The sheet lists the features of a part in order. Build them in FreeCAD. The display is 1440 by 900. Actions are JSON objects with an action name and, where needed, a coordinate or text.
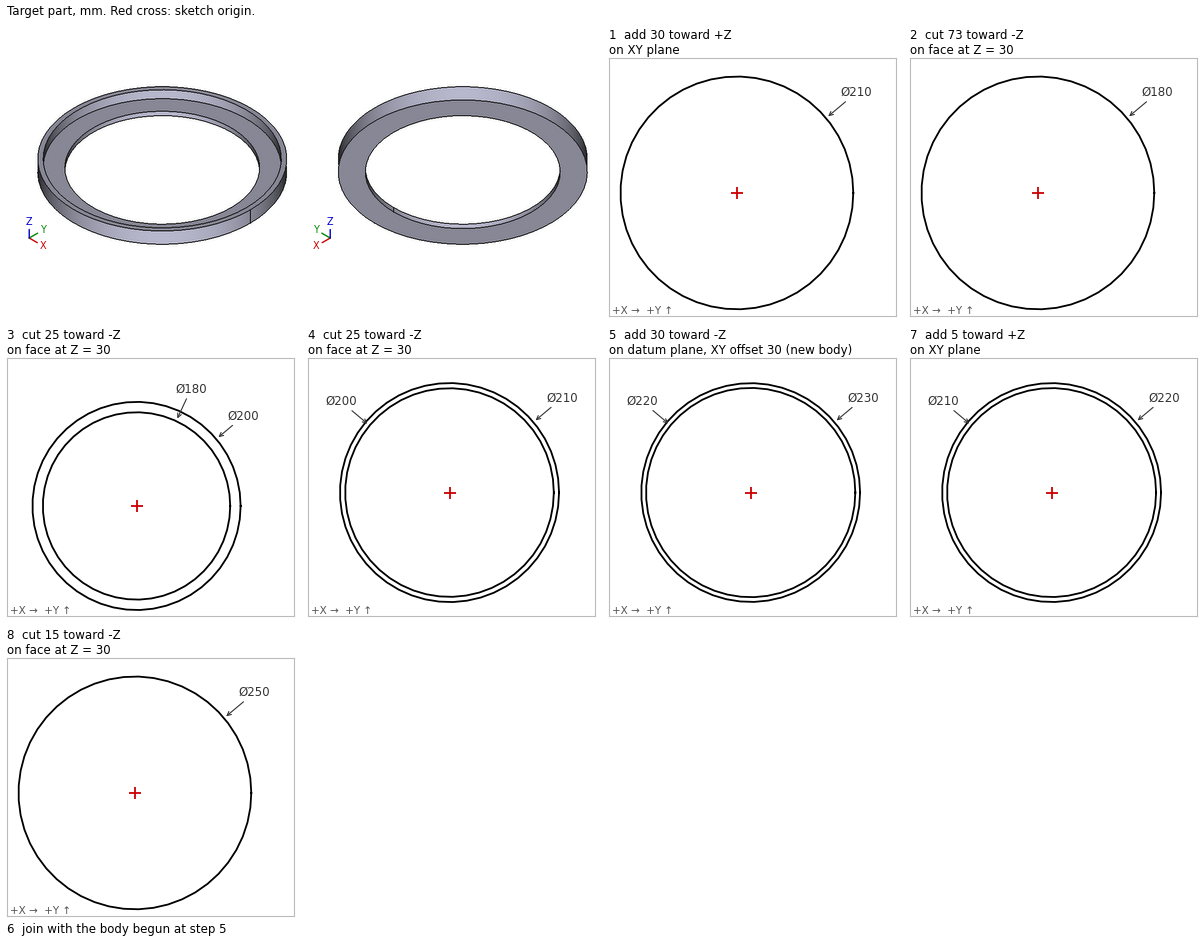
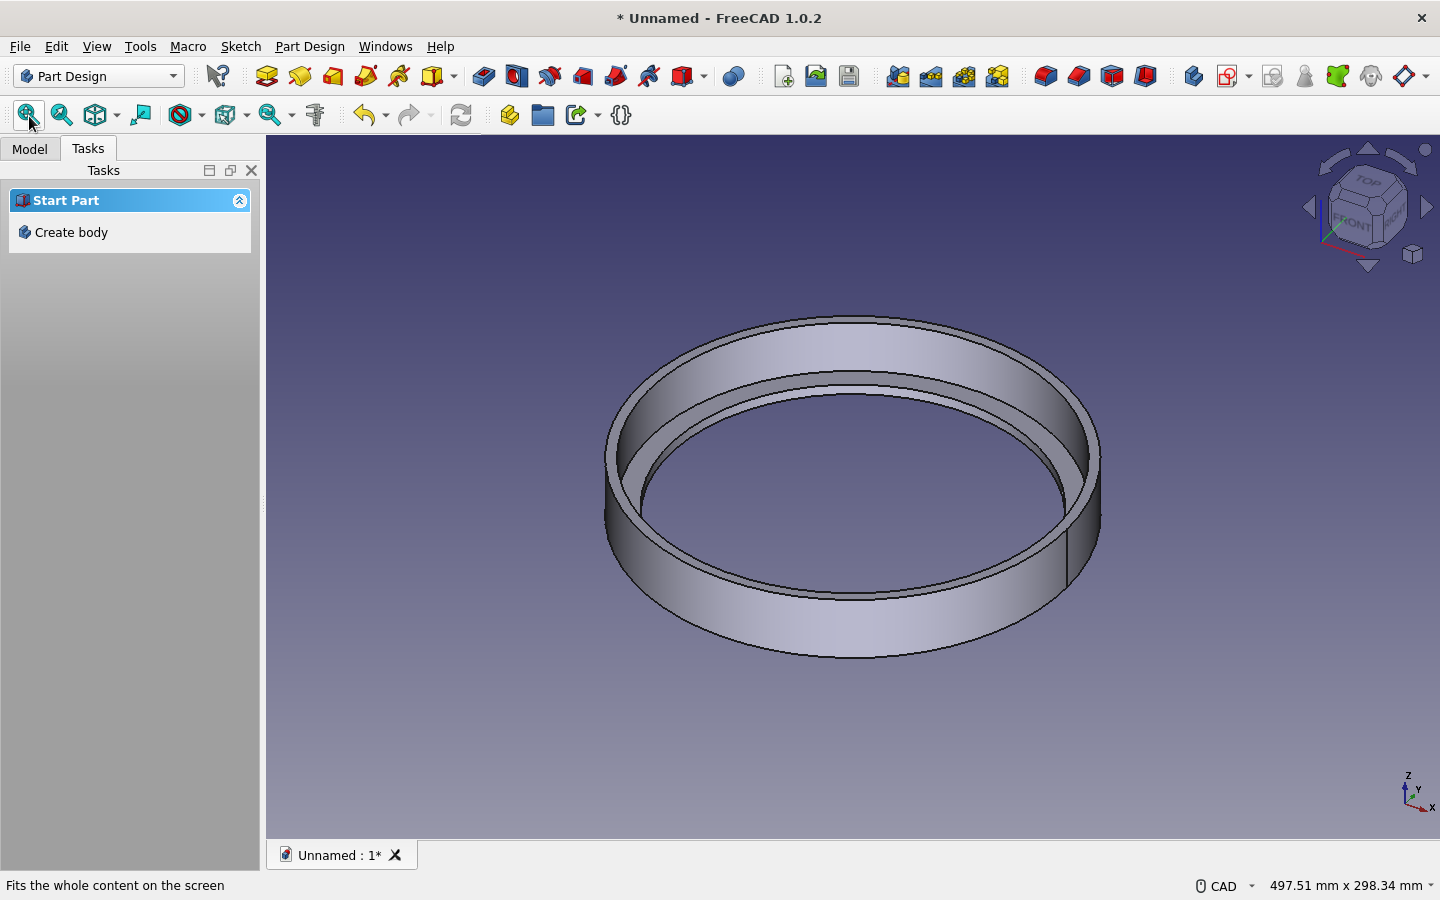
{"action": "key", "text": "0"}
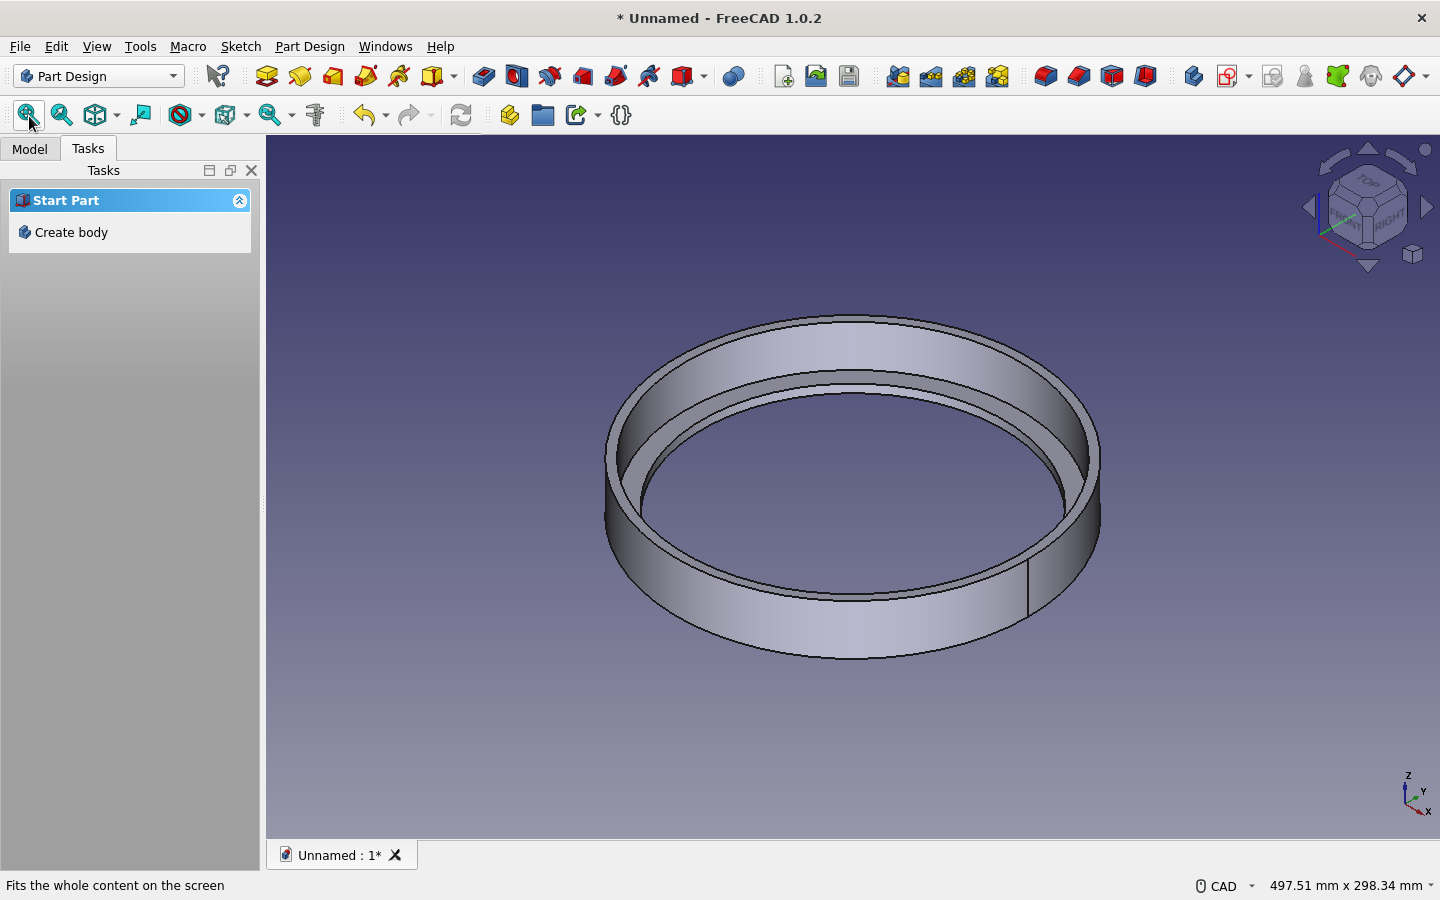
{"action": "scroll", "coordinate": [730, 579], "scroll_direction": "up", "scroll_amount": 6}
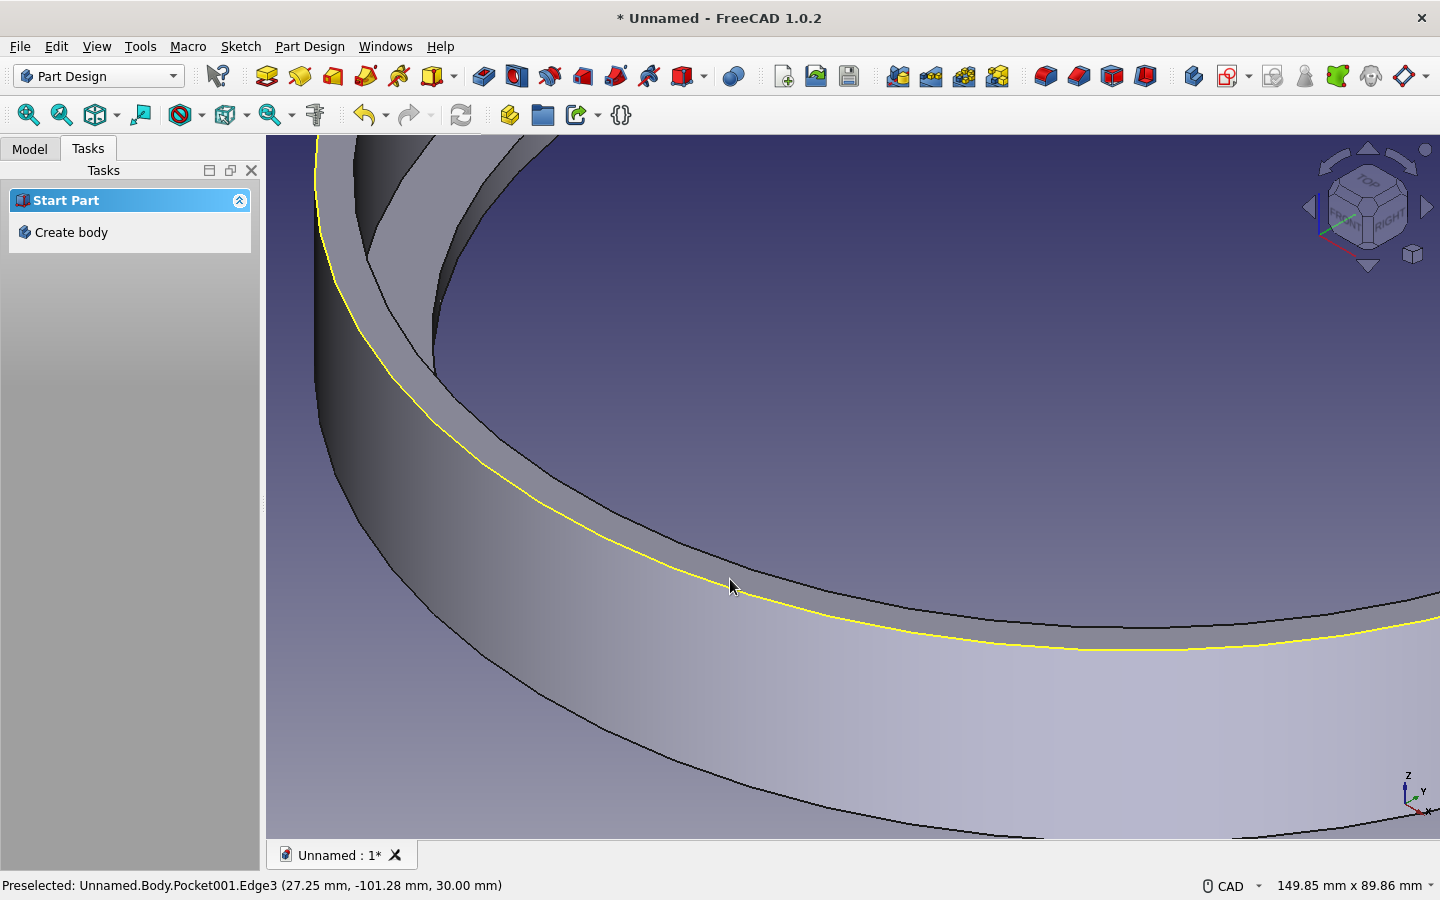
{"action": "left_click", "coordinate": [406, 376]}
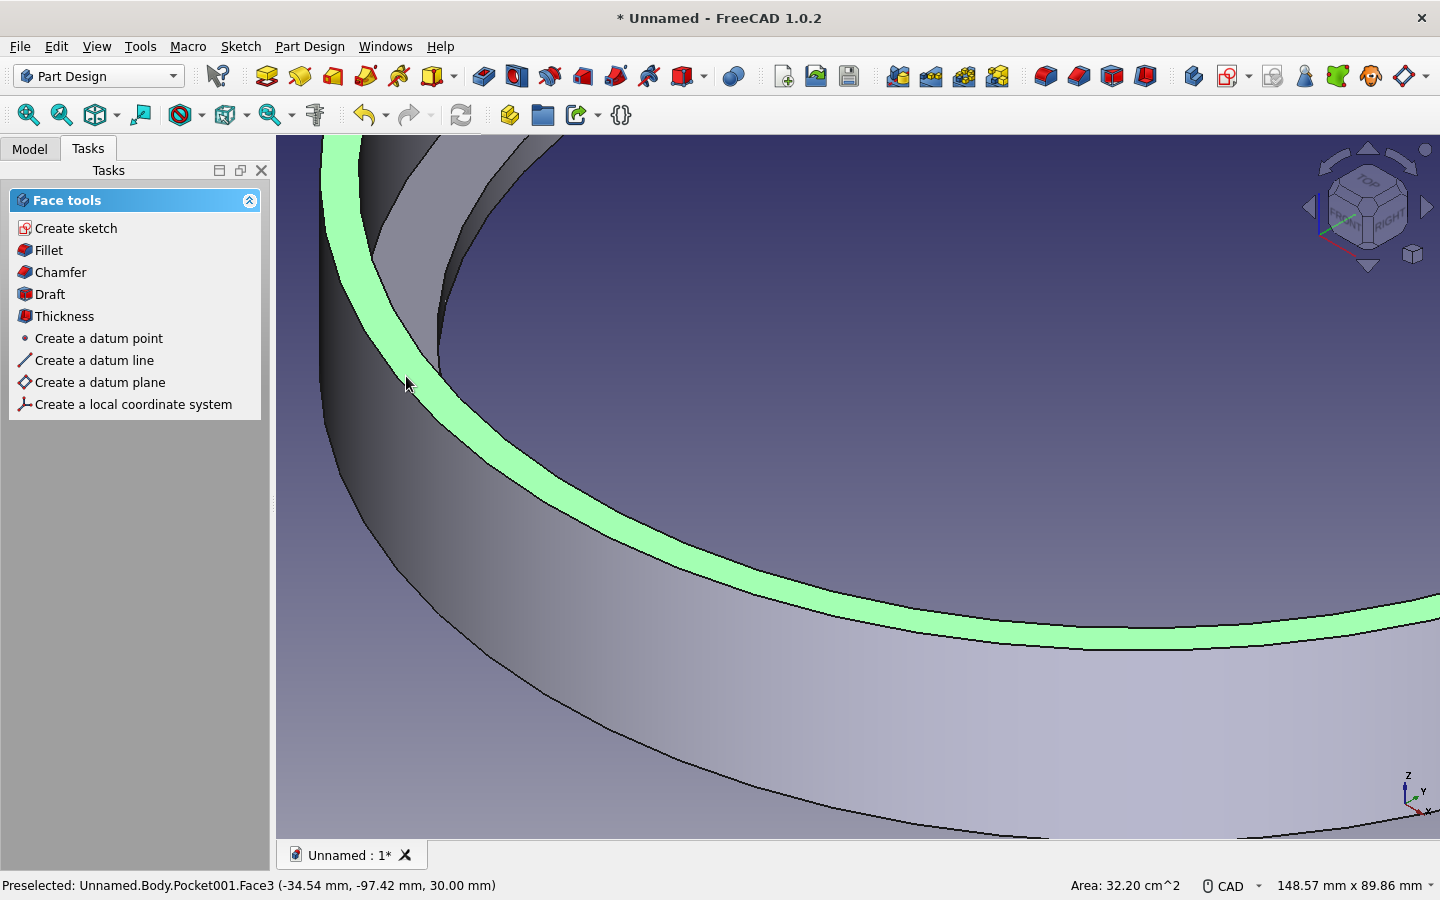
{"action": "left_click", "coordinate": [1226, 76]}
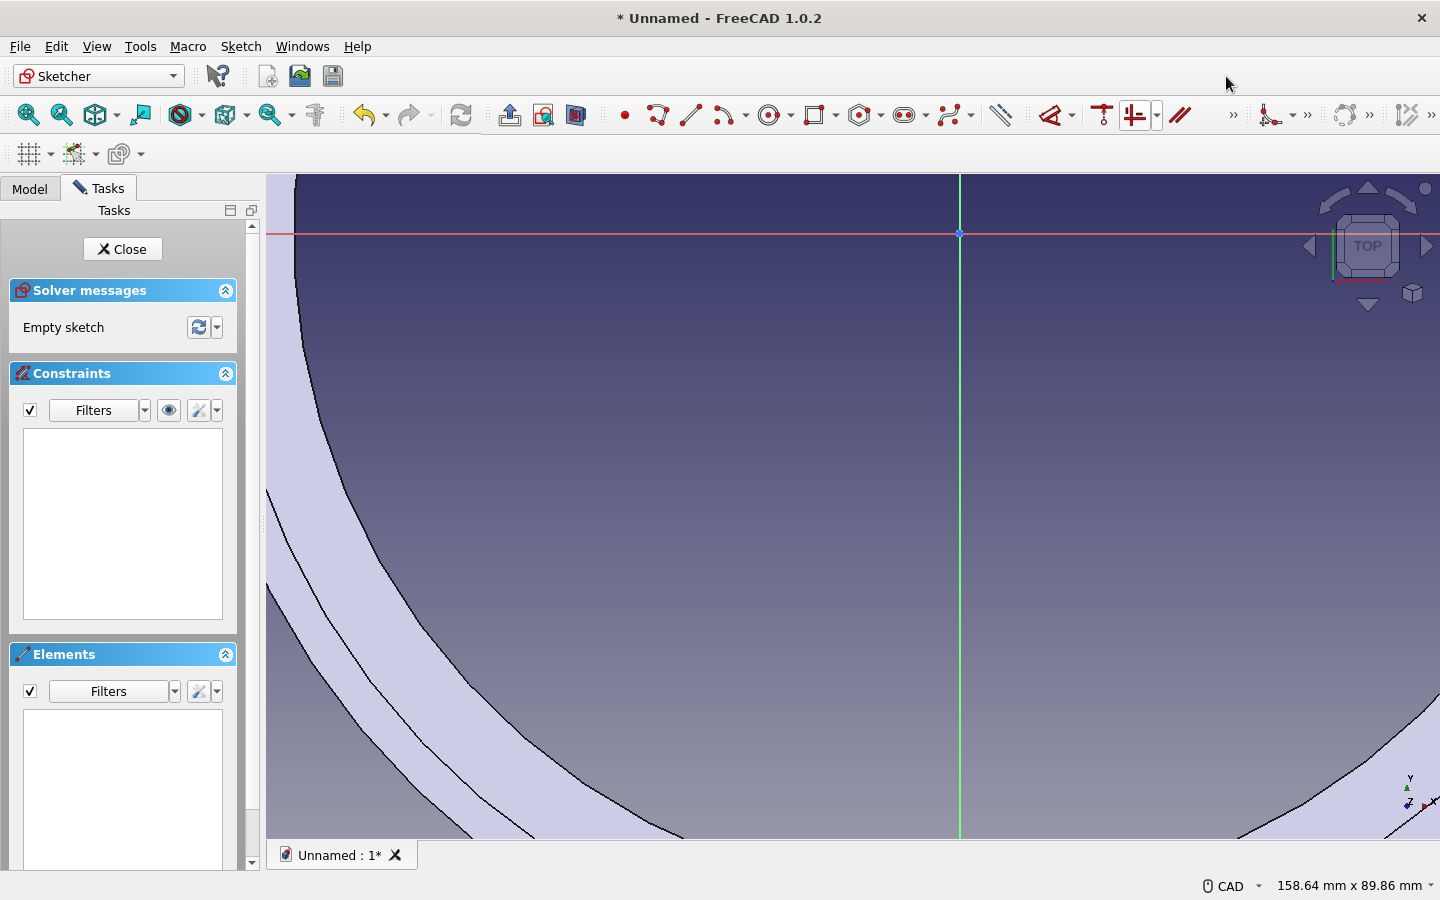
{"action": "scroll", "coordinate": [709, 624], "scroll_direction": "down", "scroll_amount": 6}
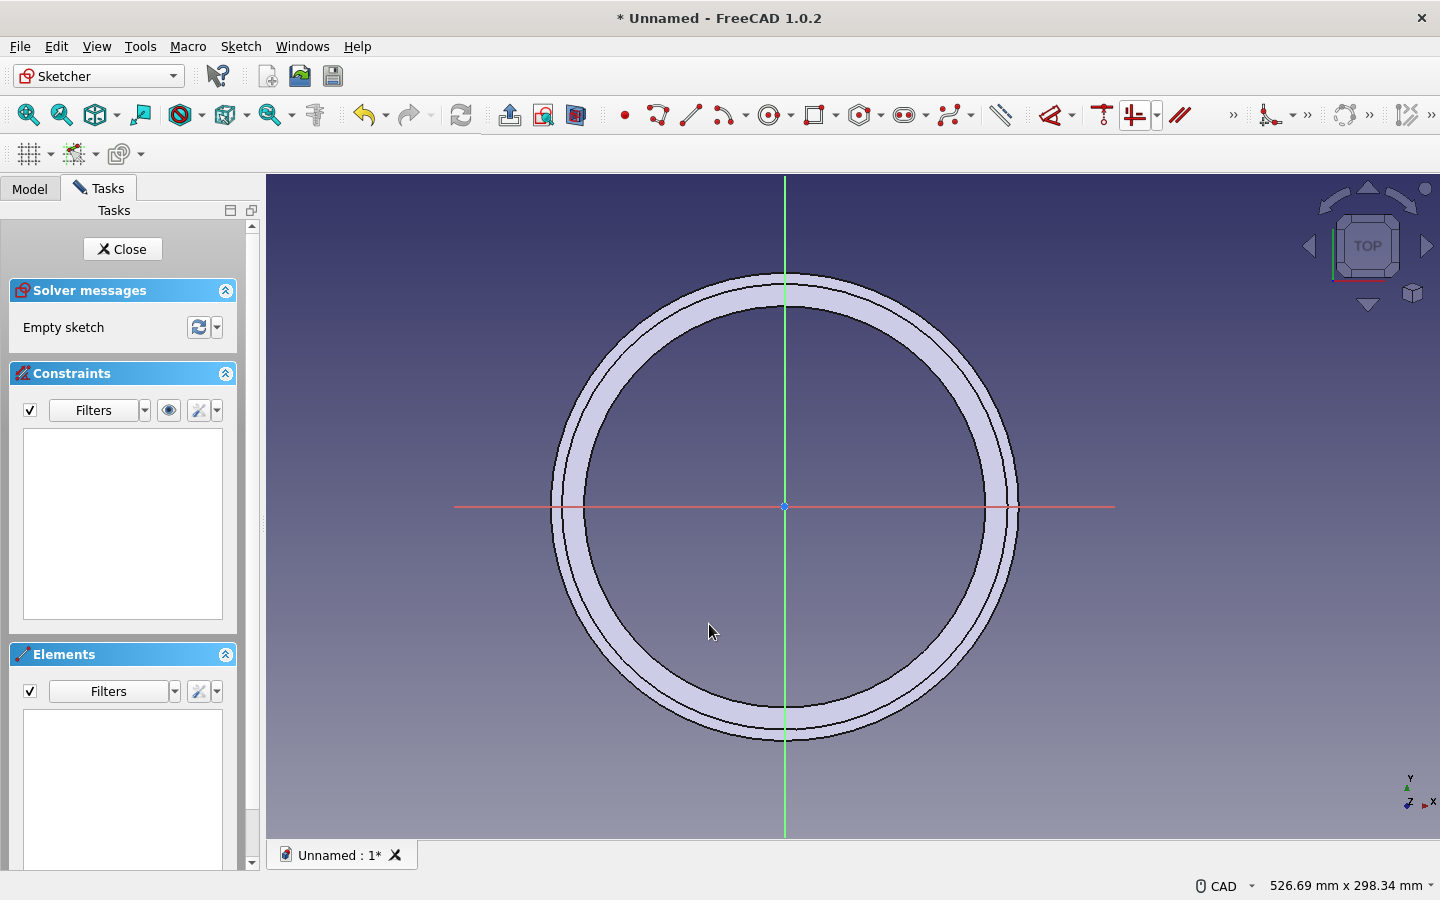
{"action": "left_click", "coordinate": [768, 116]}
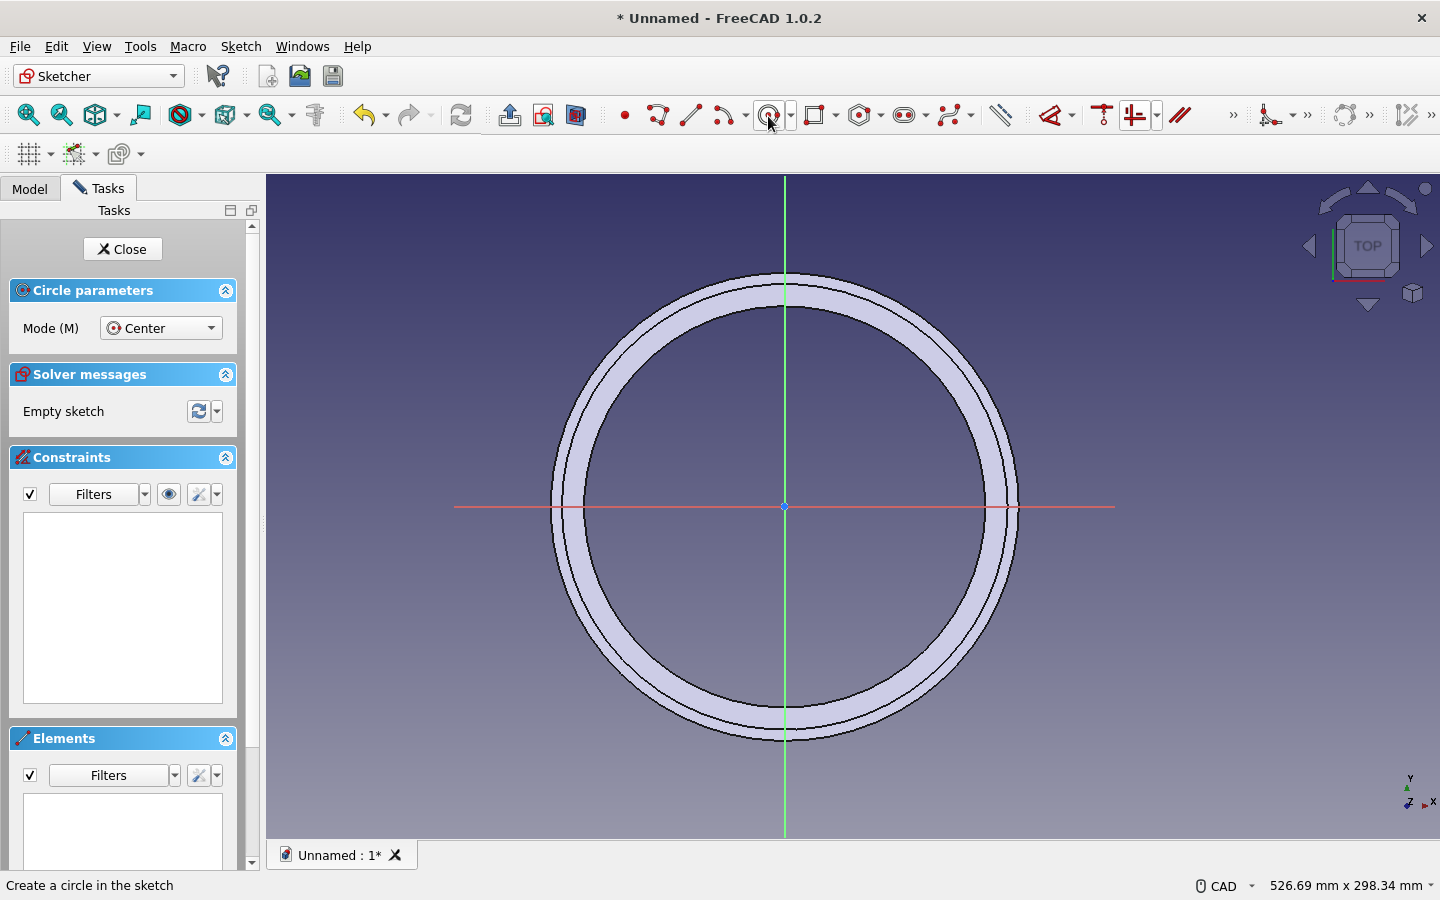
{"action": "left_click", "coordinate": [785, 507]}
{"action": "mouse_move", "coordinate": [950, 341]}